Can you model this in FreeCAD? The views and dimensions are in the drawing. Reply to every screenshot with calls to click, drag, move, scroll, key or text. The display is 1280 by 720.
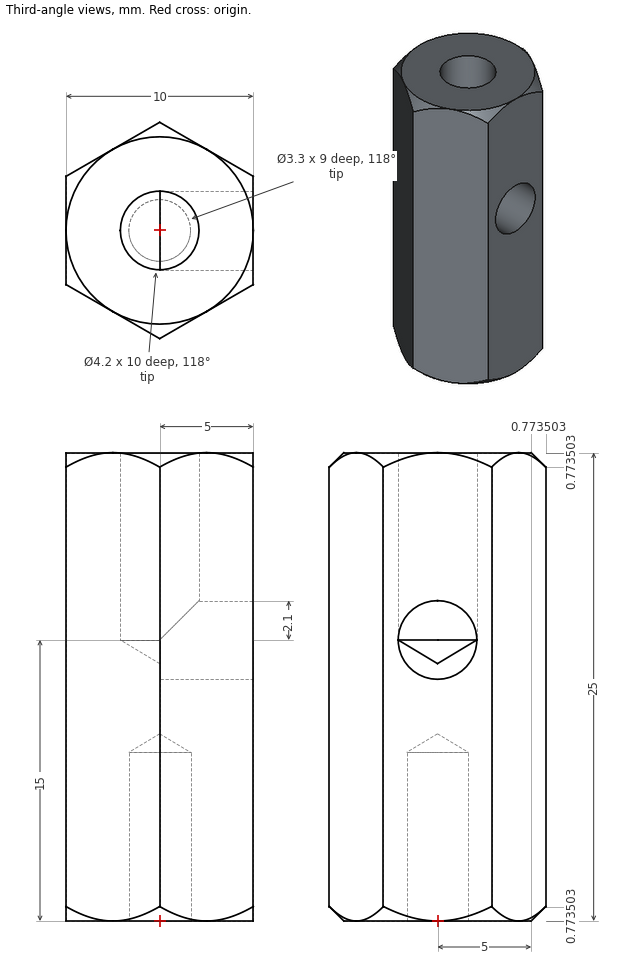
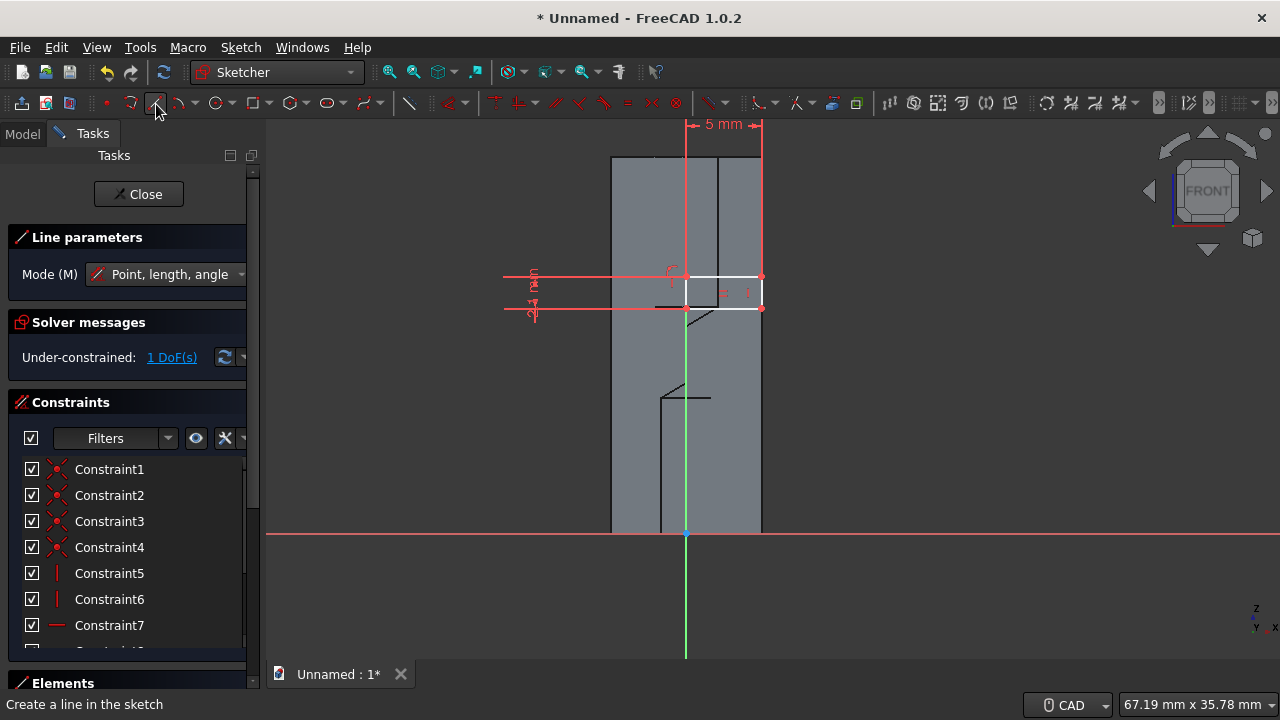
scroll(769, 307, up, 4)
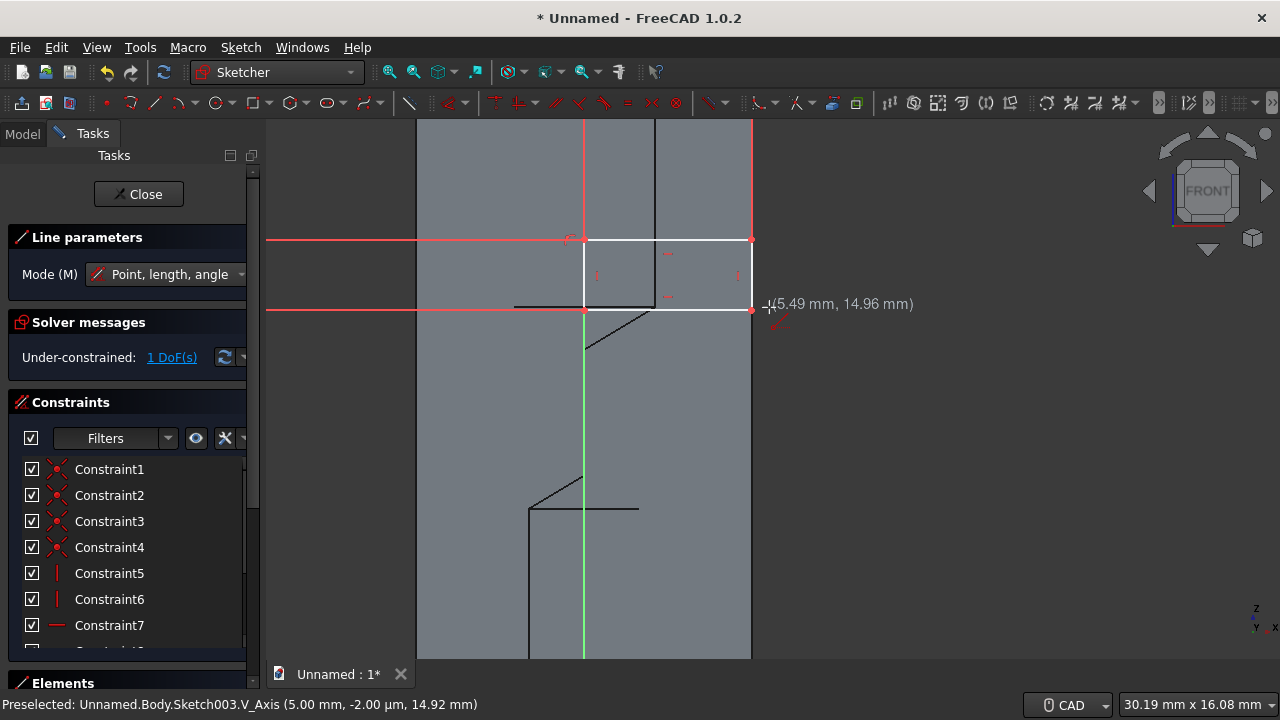
click(769, 307)
click(819, 307)
key(Escape)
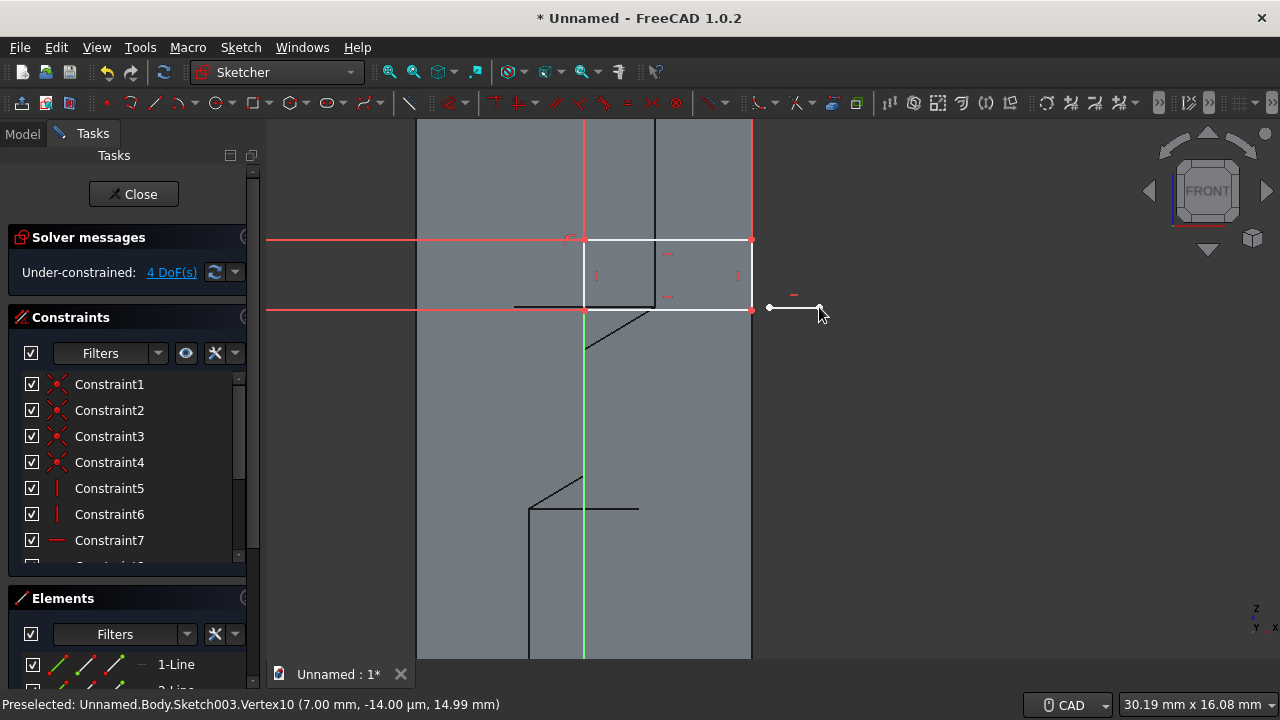
click(784, 308)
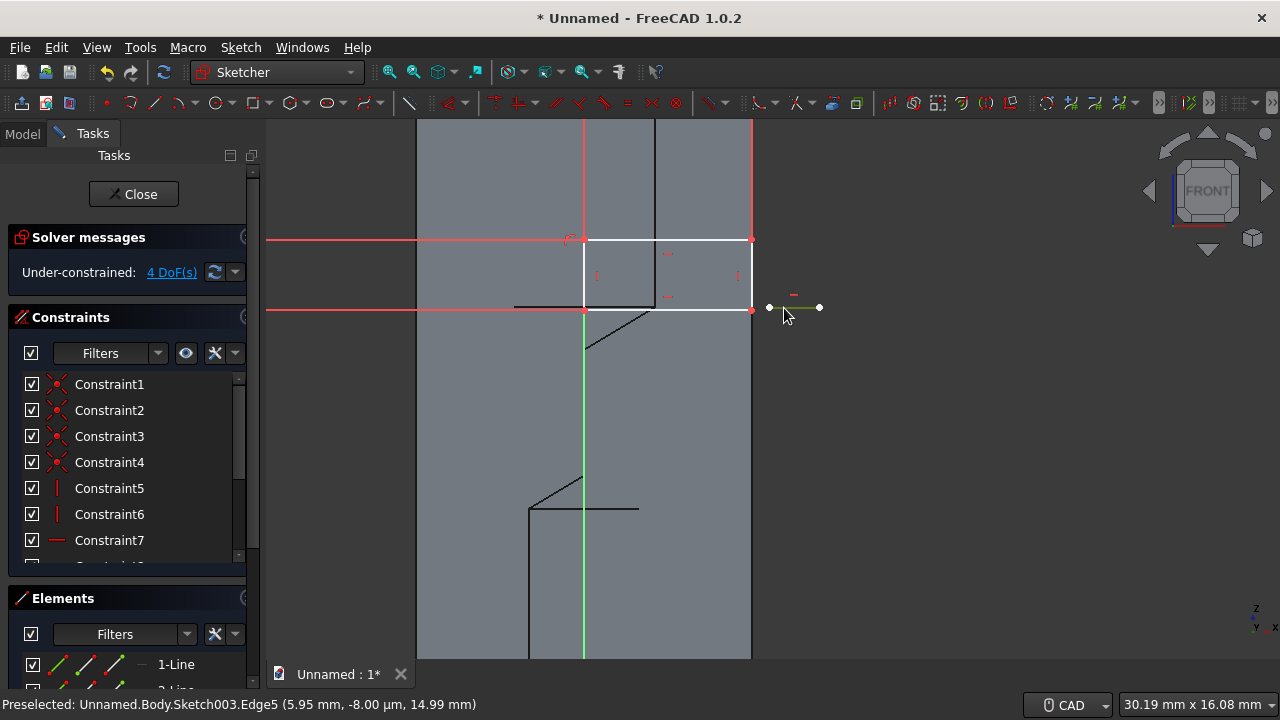
click(410, 104)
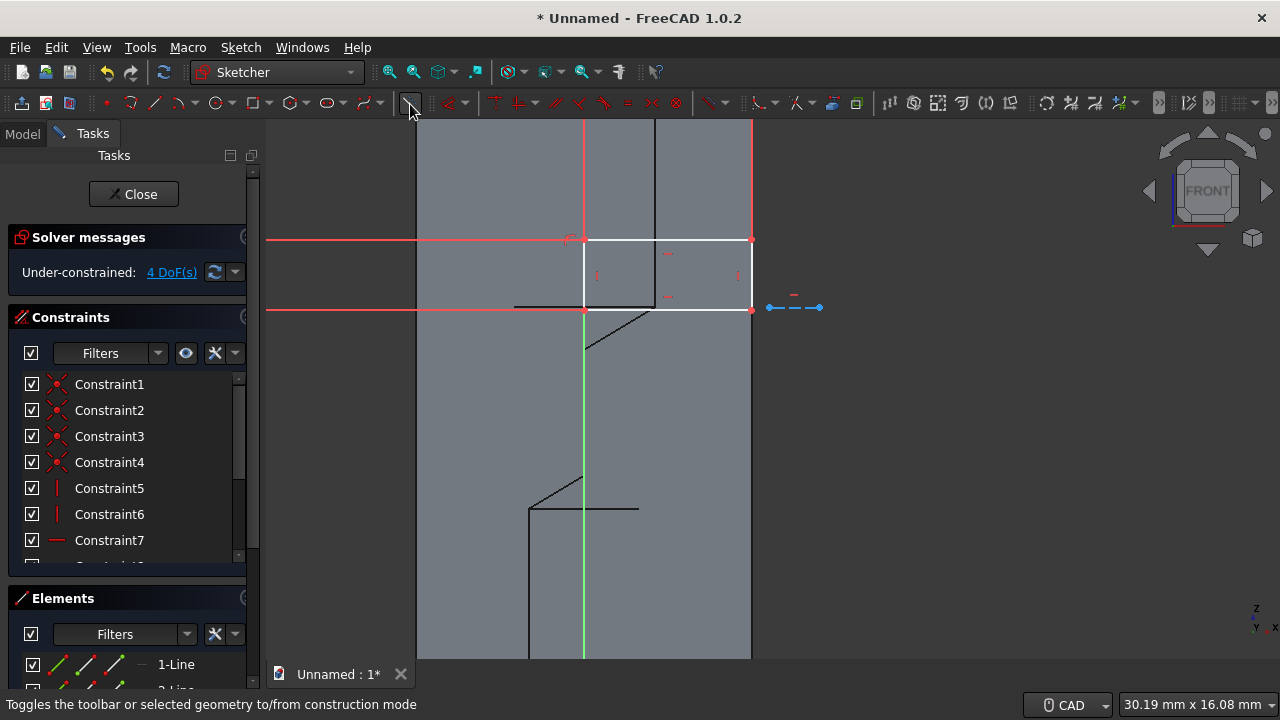
key(d)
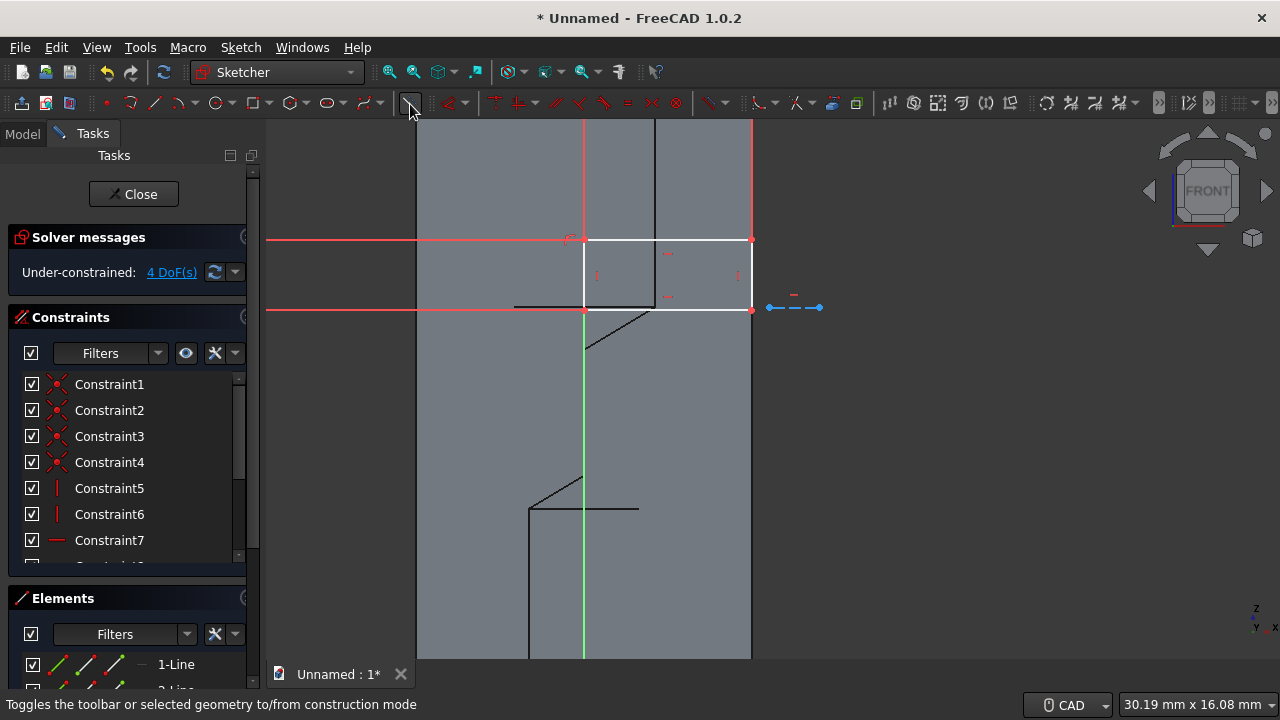
click(584, 310)
click(550, 471)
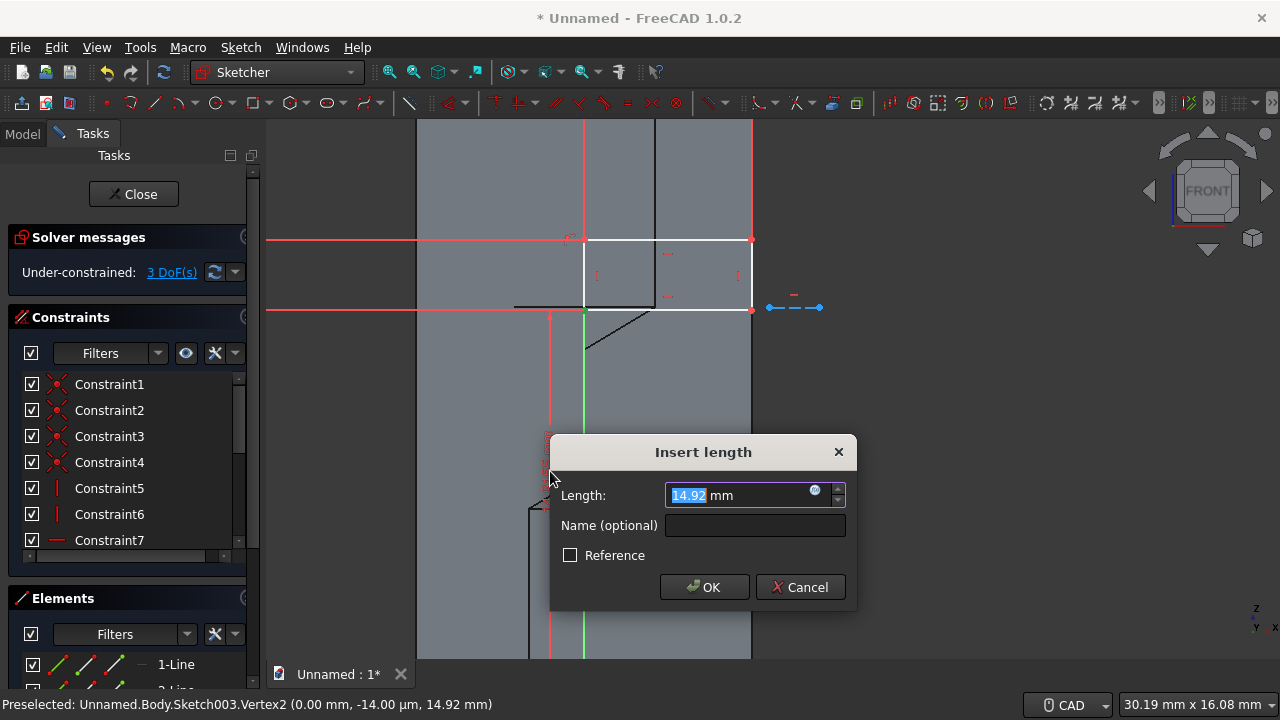
text(15)
key(Return)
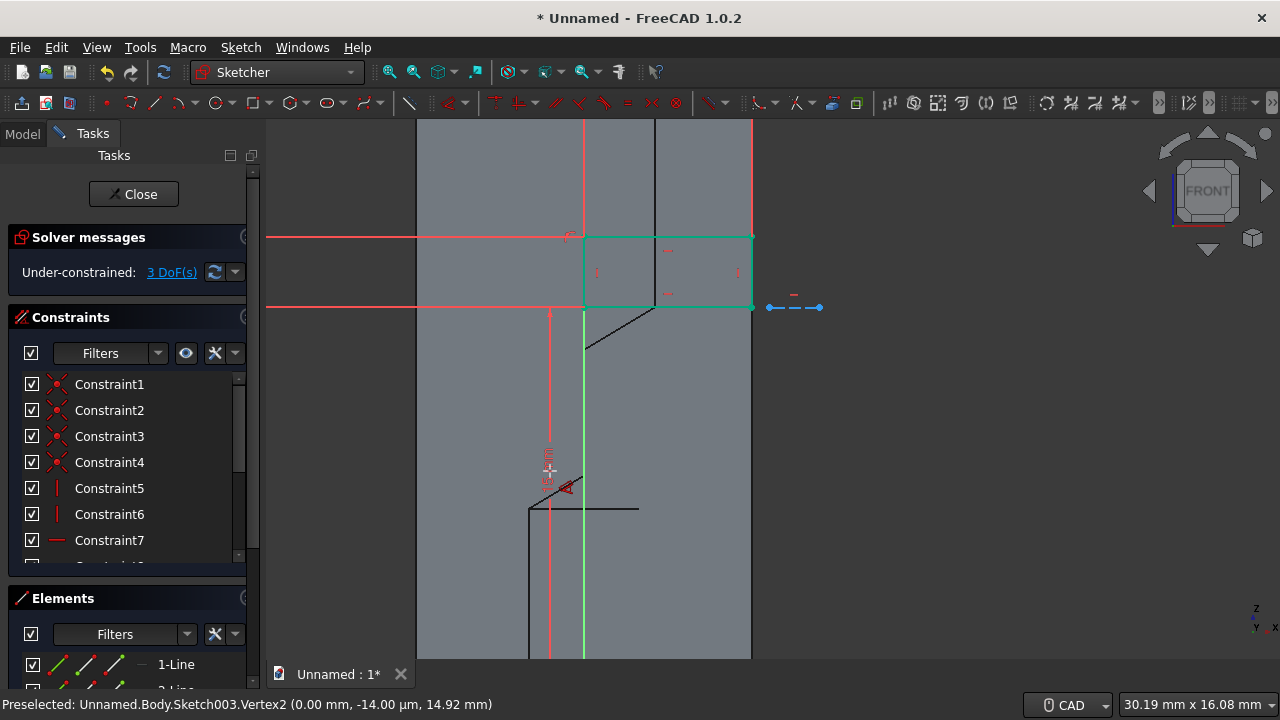
click(769, 308)
click(550, 395)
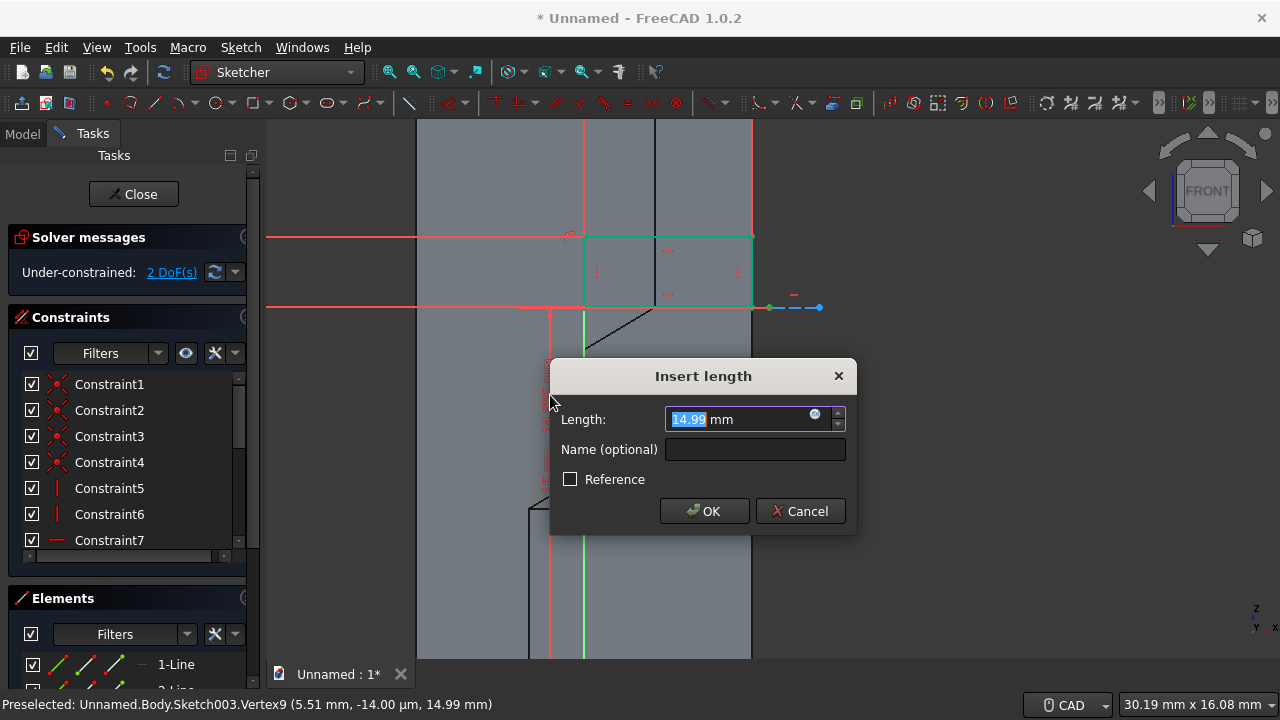
text(15)
key(Return)
key(Escape)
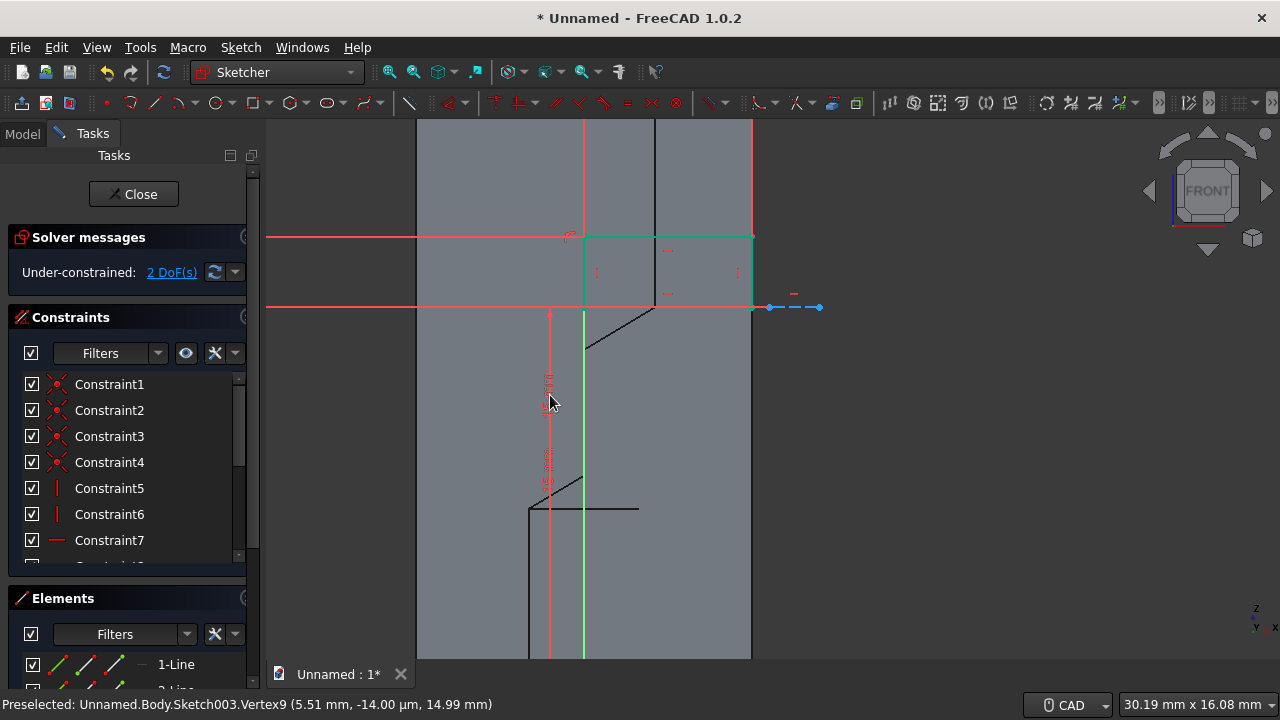
click(134, 194)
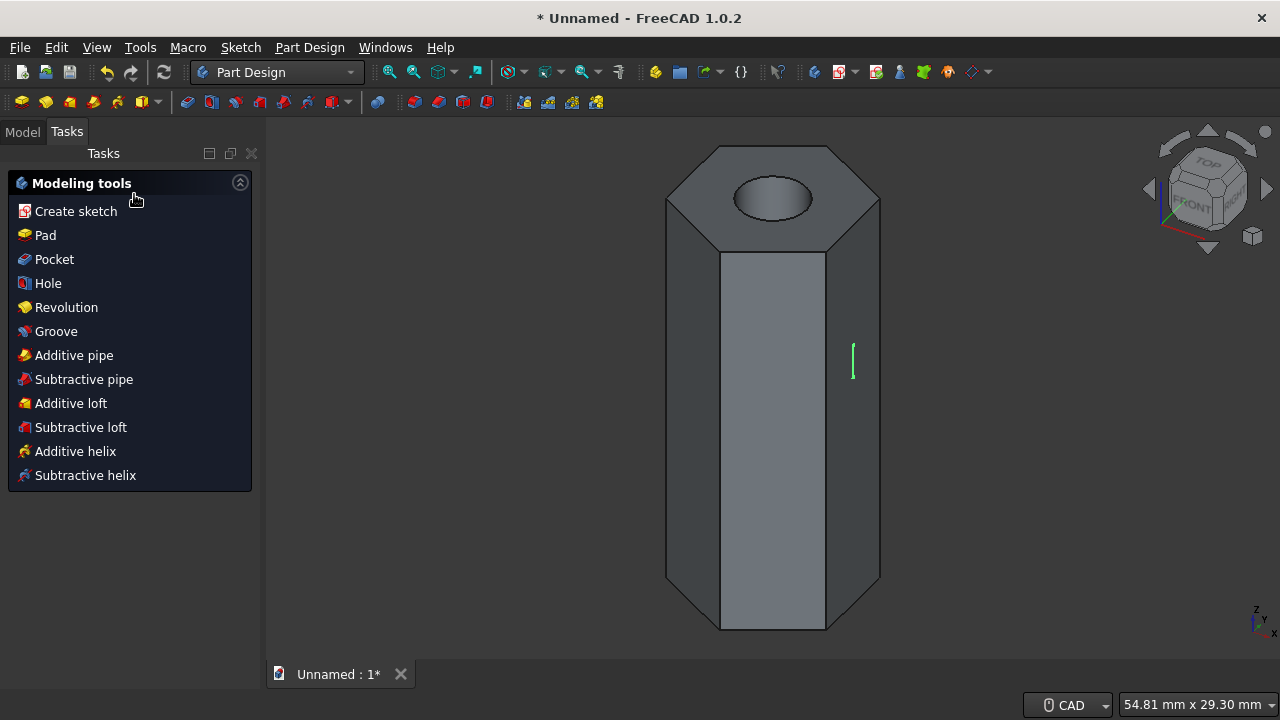
click(236, 102)